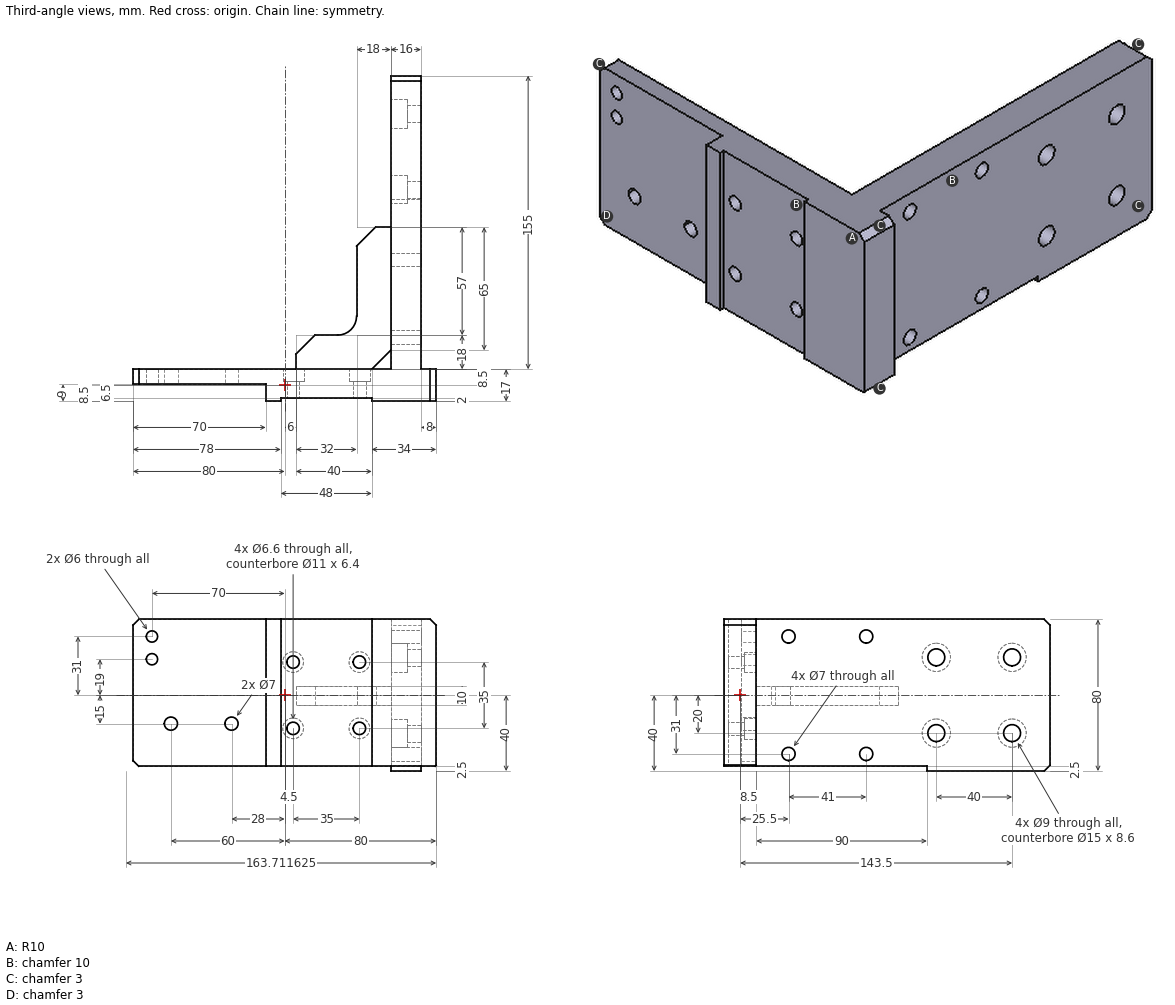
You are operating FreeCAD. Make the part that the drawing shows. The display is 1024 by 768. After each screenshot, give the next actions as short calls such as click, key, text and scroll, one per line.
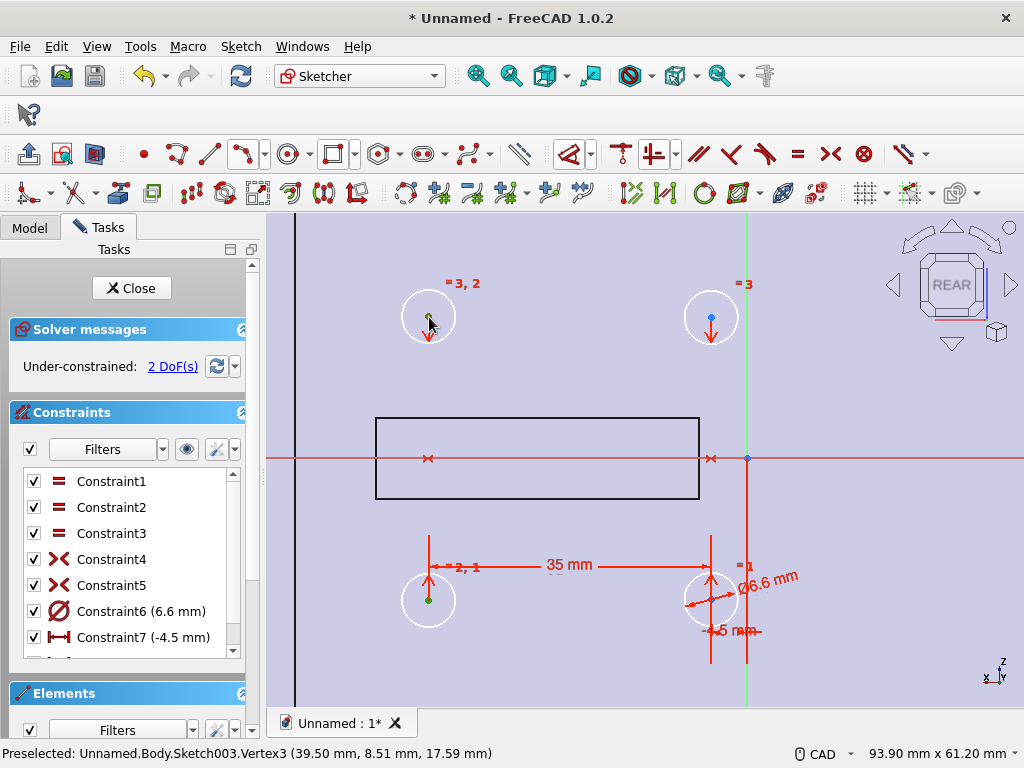
click(590, 154)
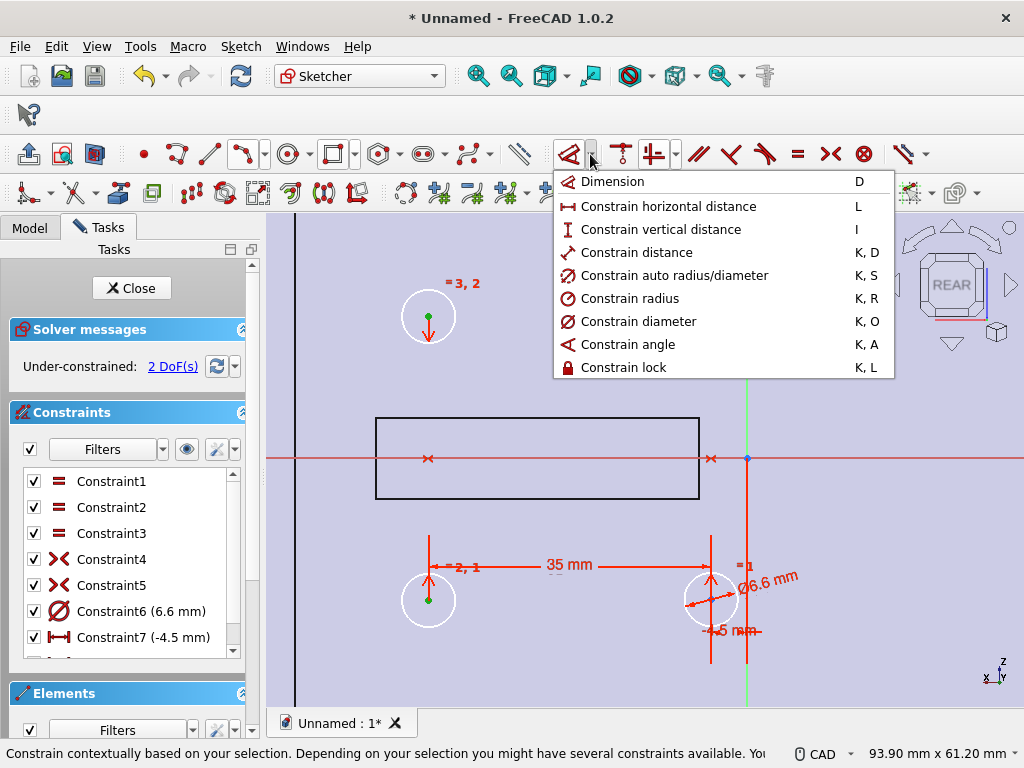
click(724, 230)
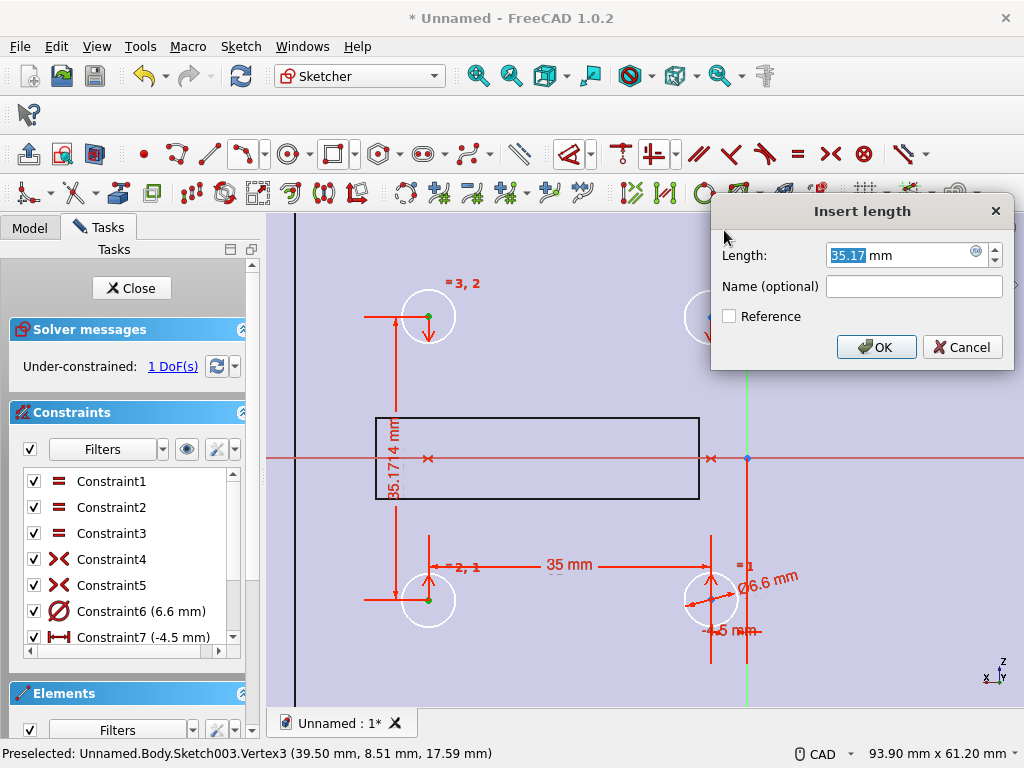
text(35)
key(Return)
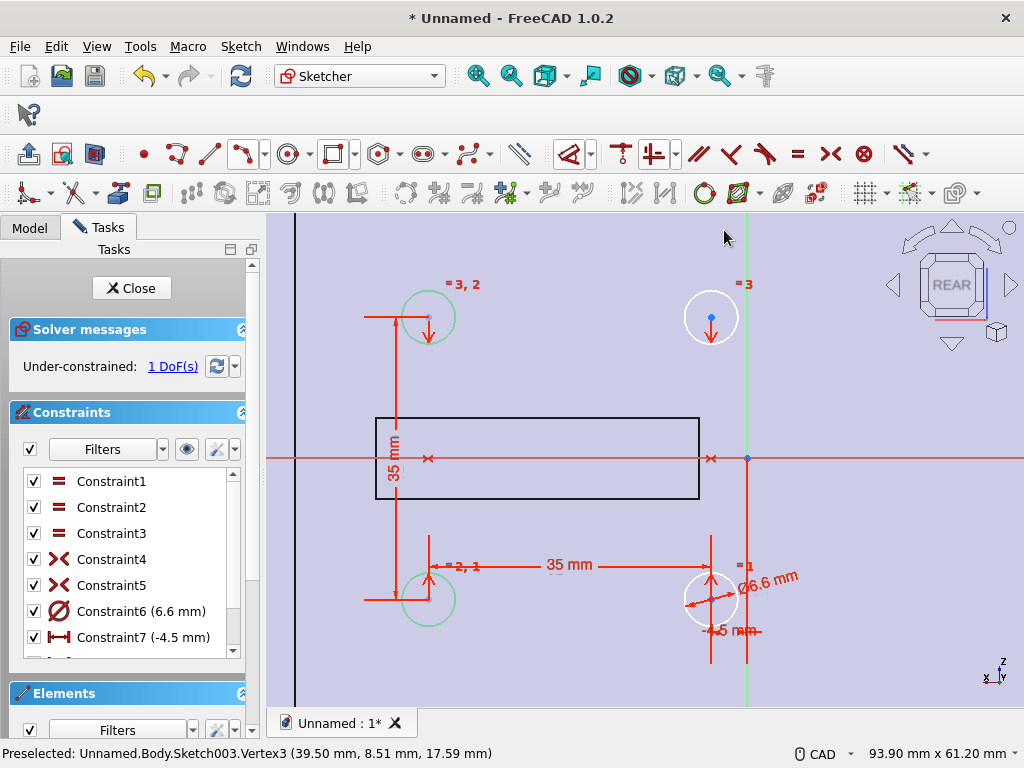
click(711, 600)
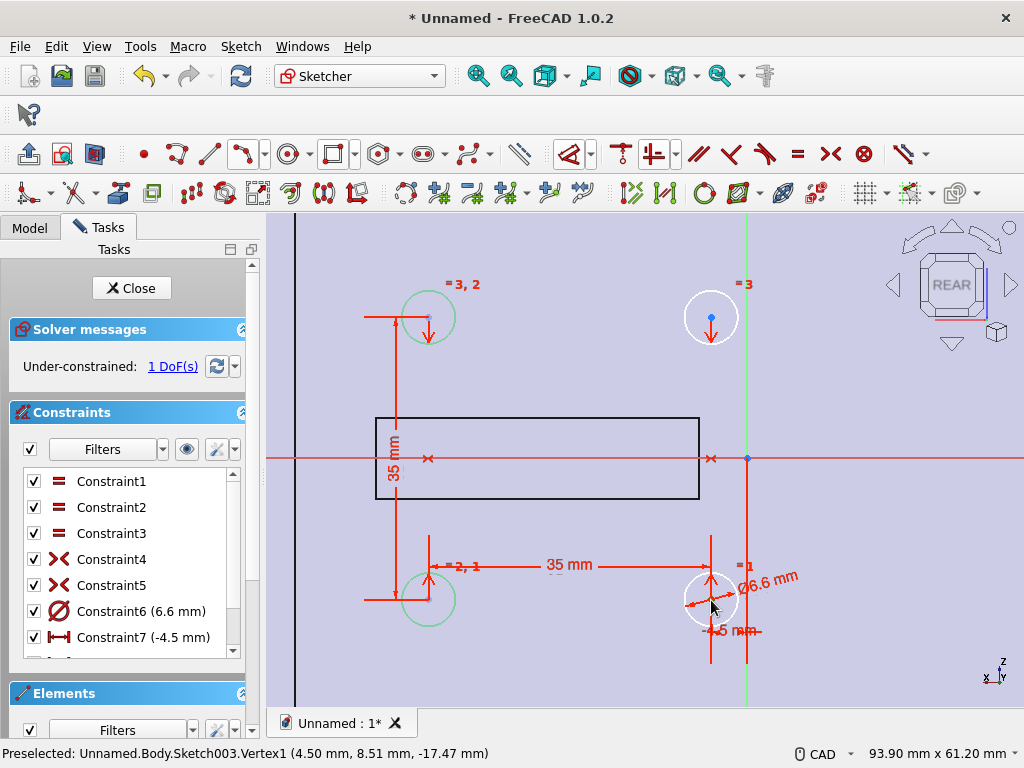
click(429, 317)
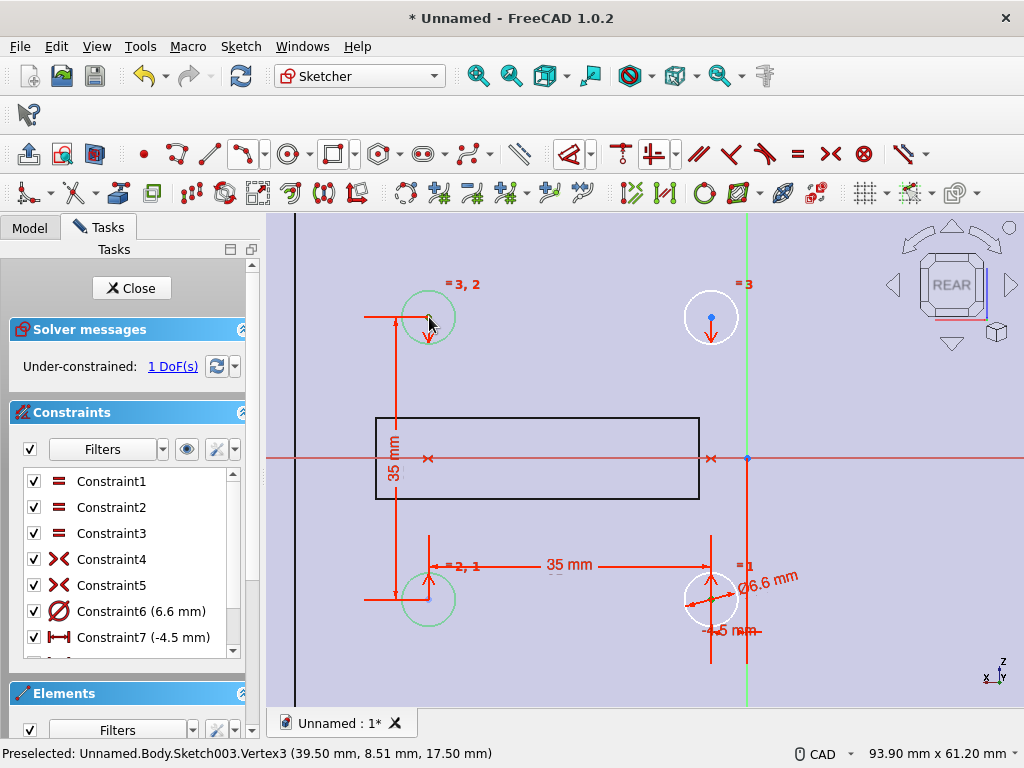
click(590, 154)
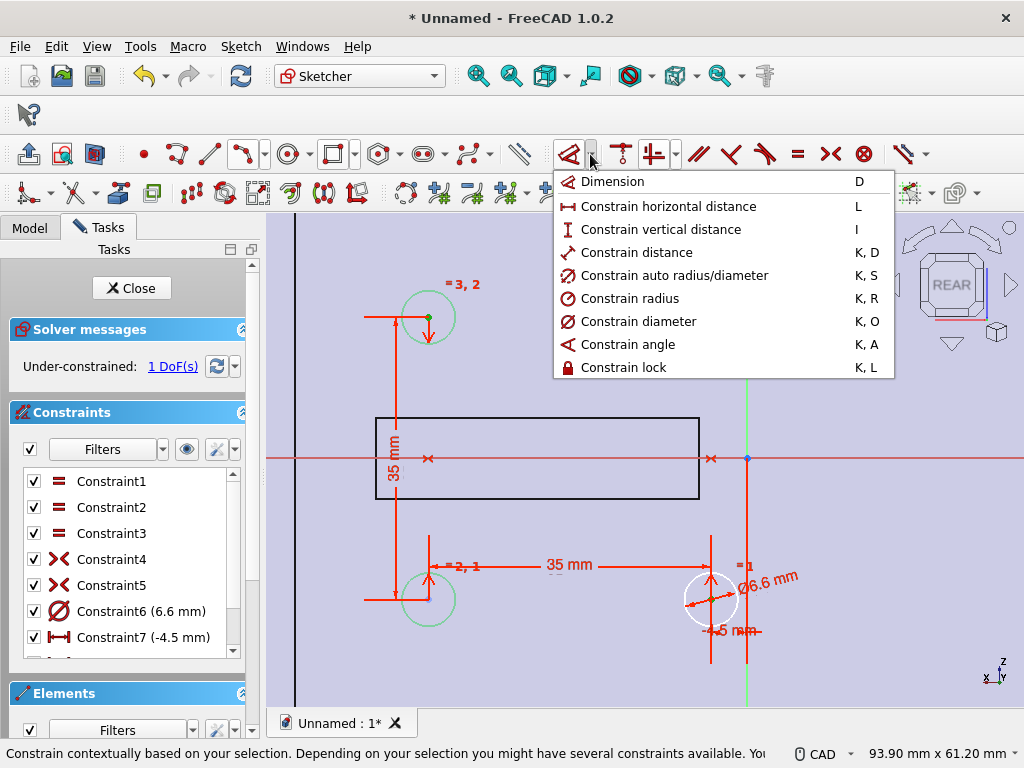
click(724, 230)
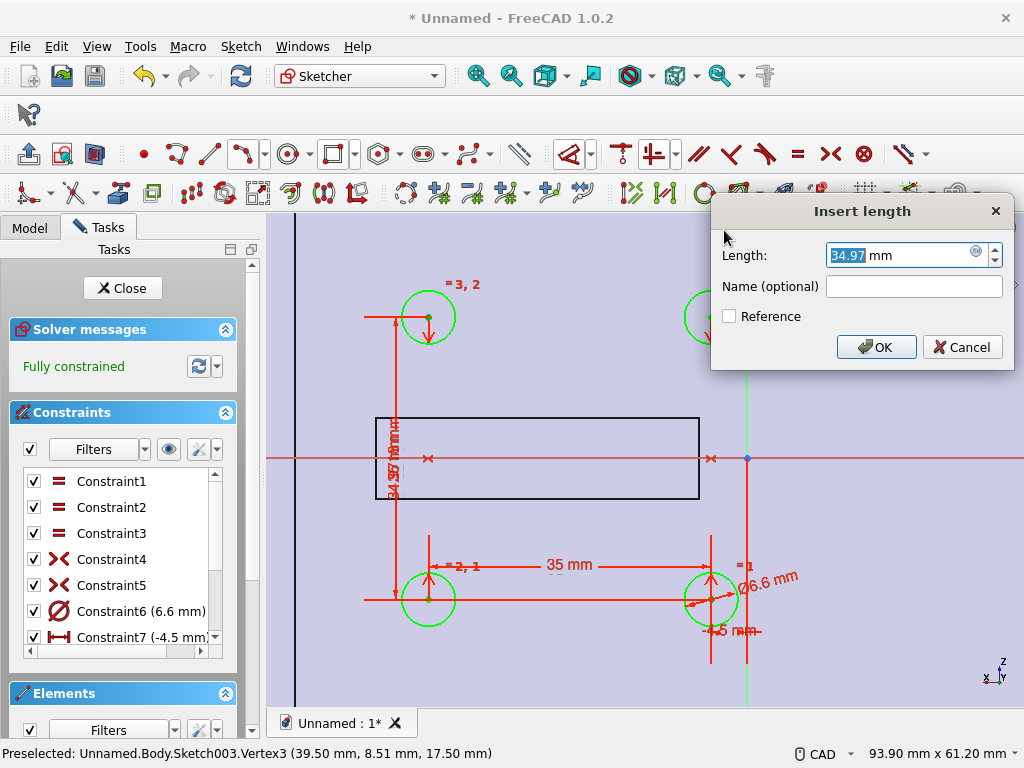
text(35)
key(Return)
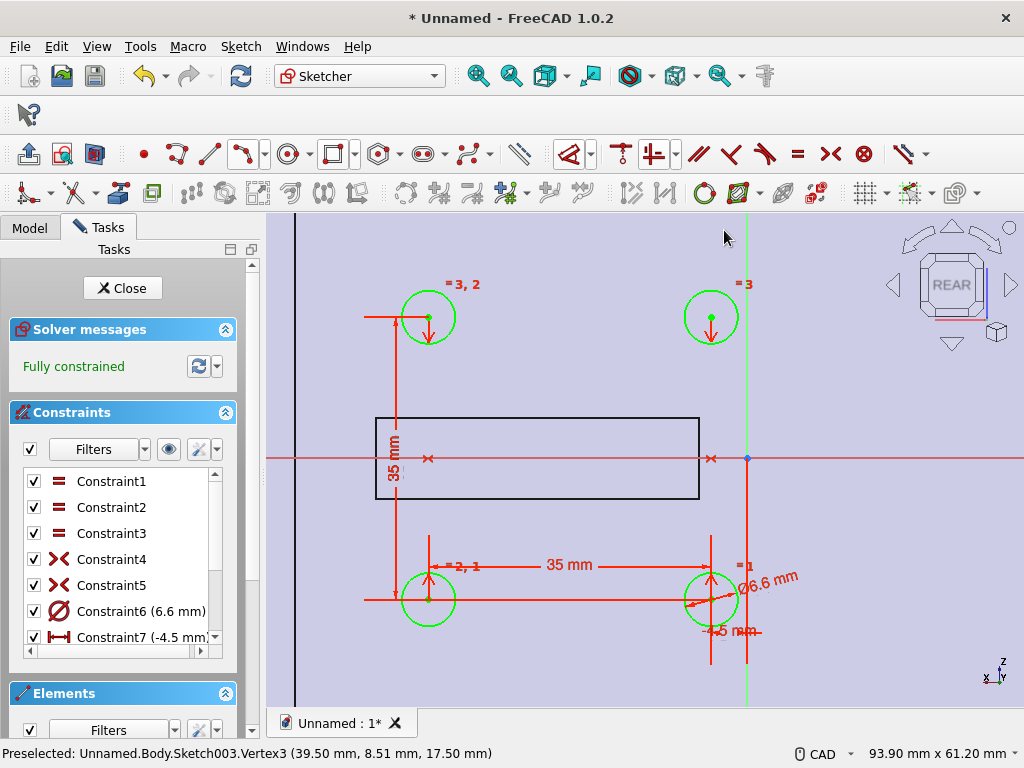
click(123, 288)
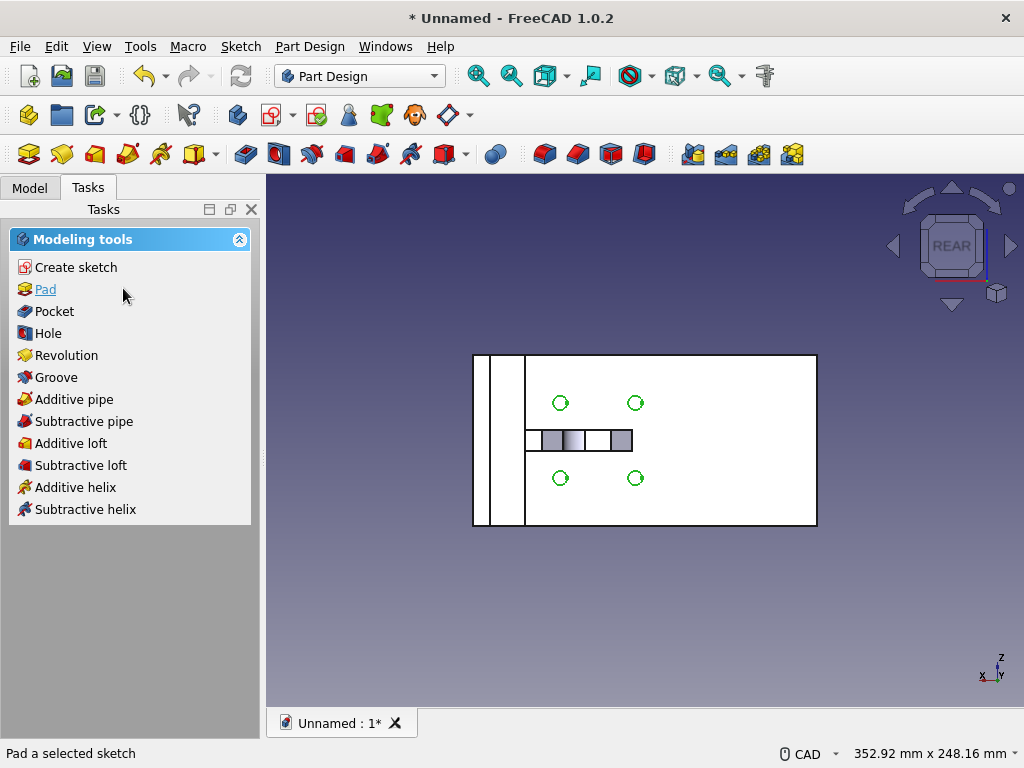
click(279, 154)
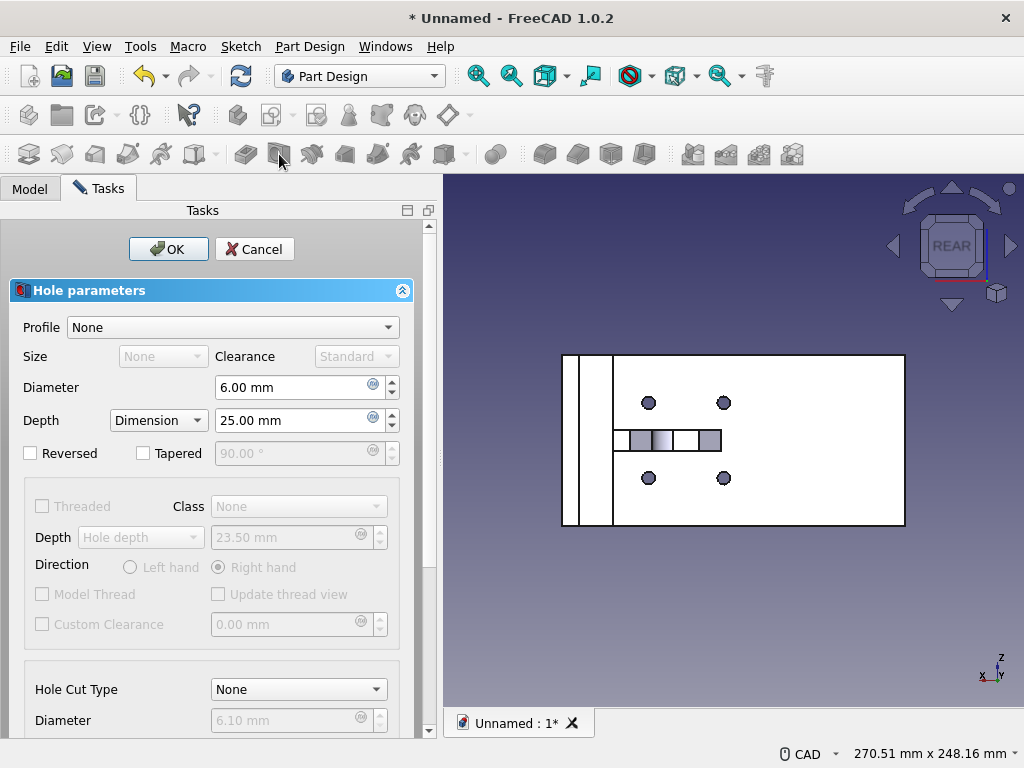
triple_click(300, 388)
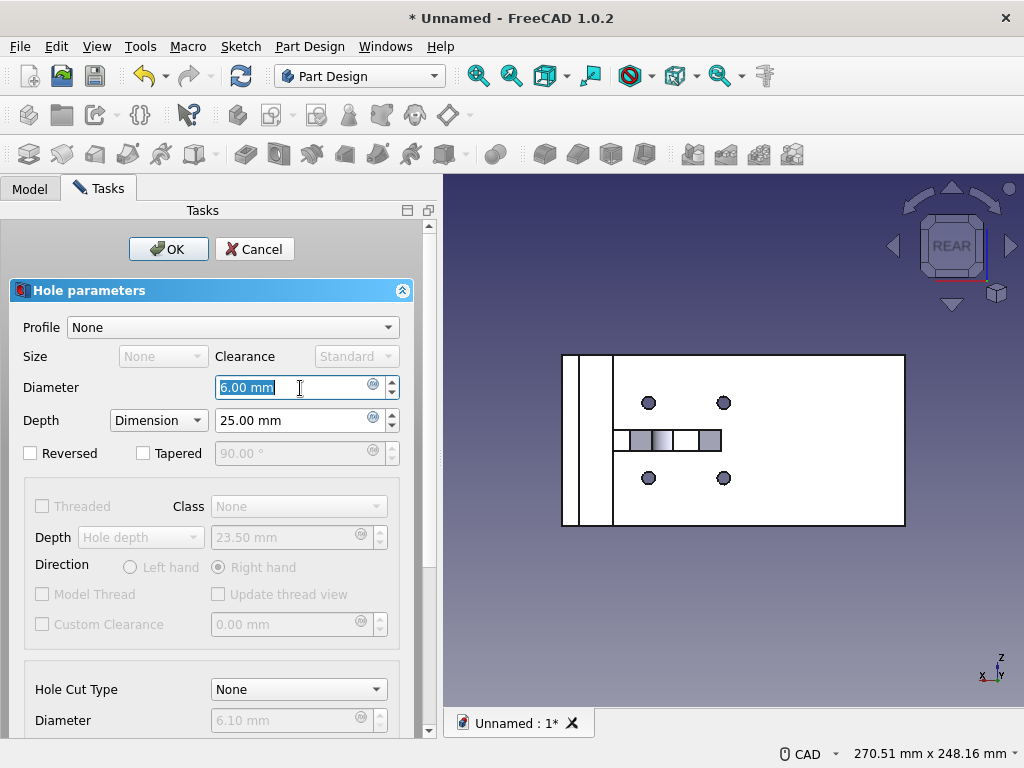
text(6.6)
key(Tab)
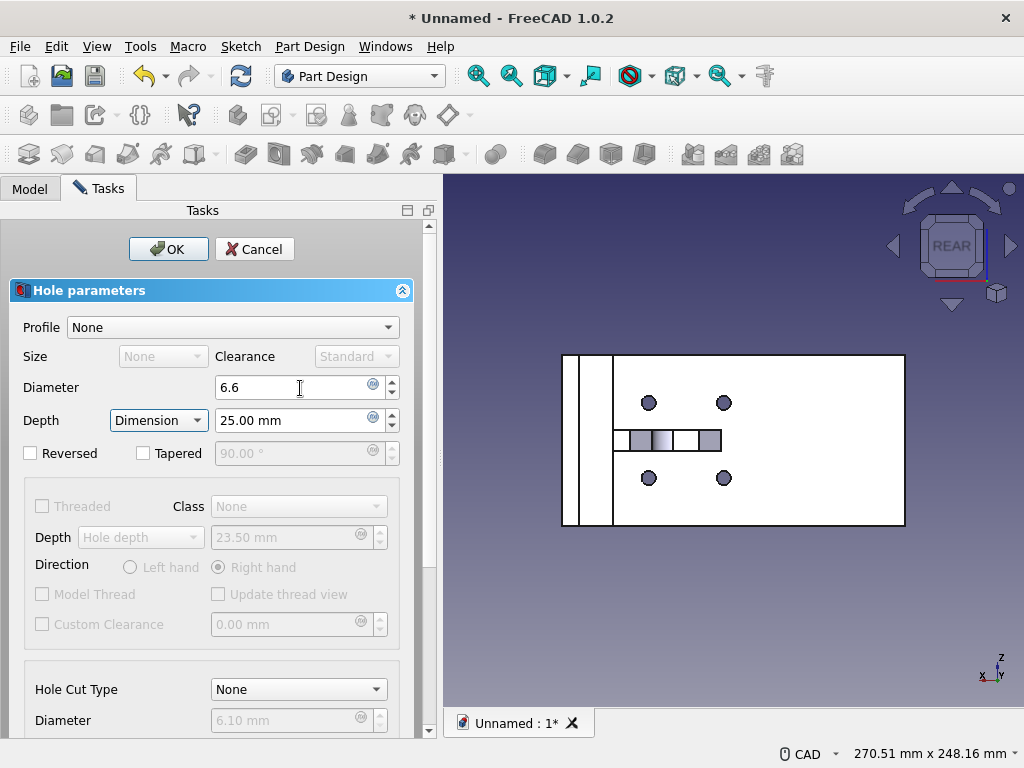
click(160, 420)